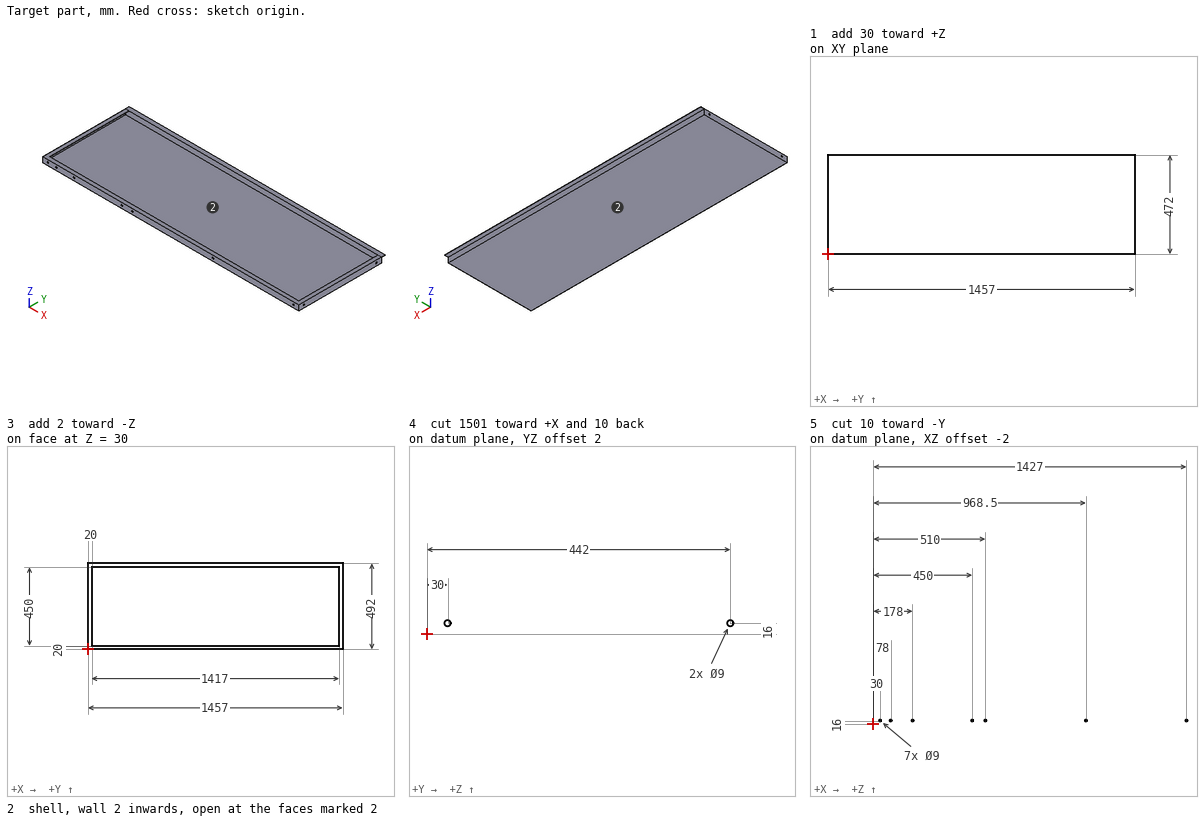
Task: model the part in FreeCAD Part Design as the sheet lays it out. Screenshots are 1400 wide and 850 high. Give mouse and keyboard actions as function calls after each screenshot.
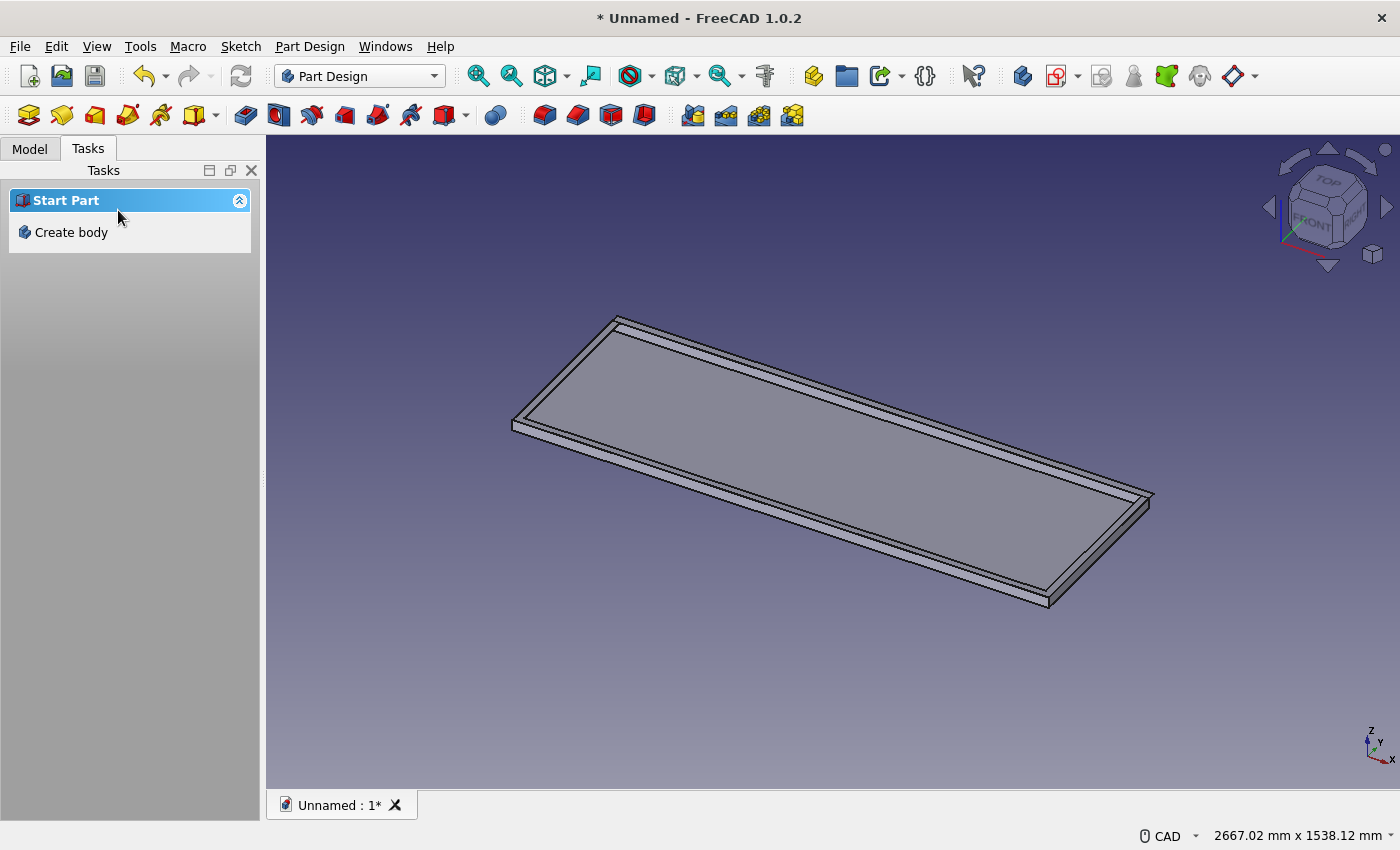
click(30, 148)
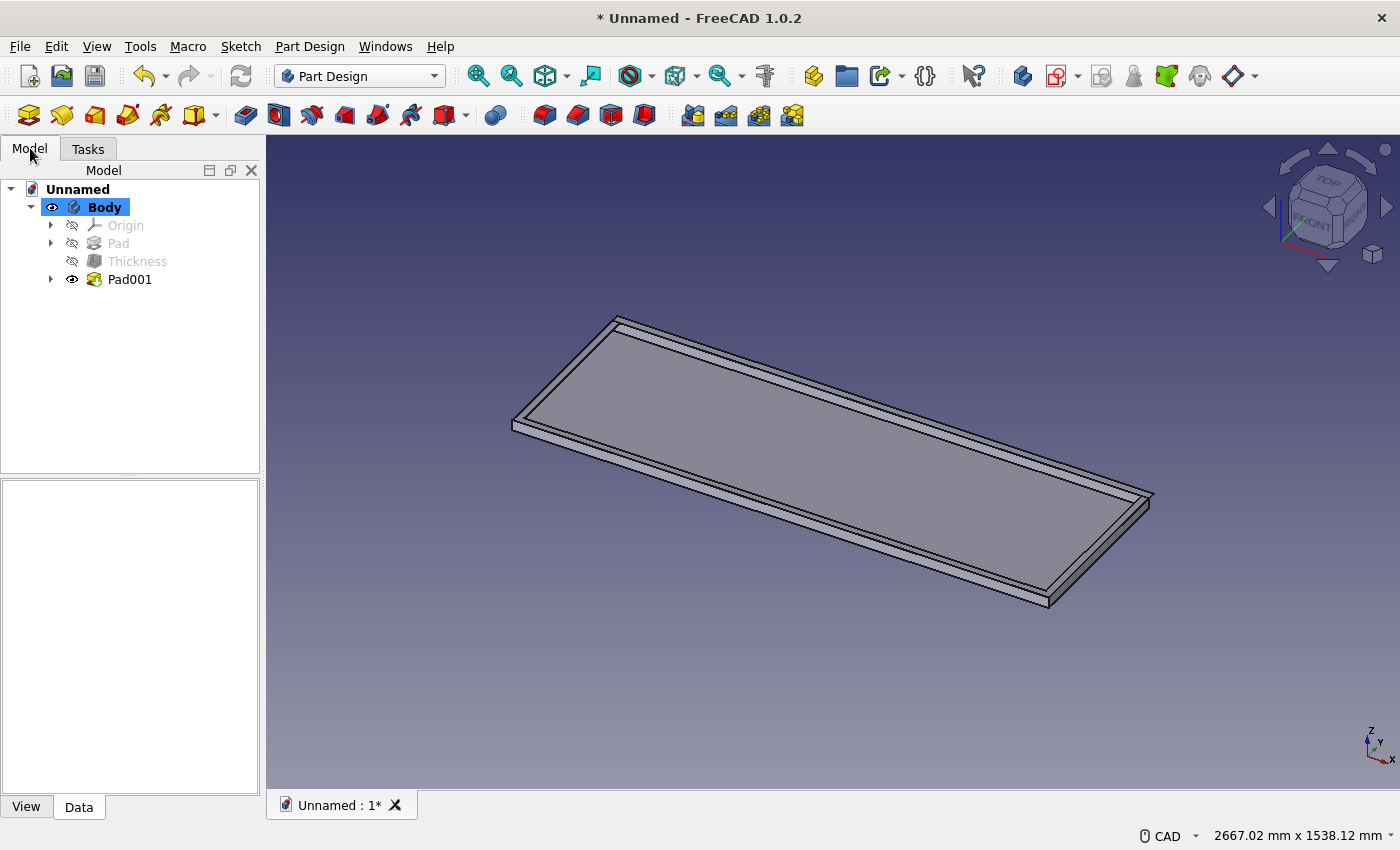
click(51, 225)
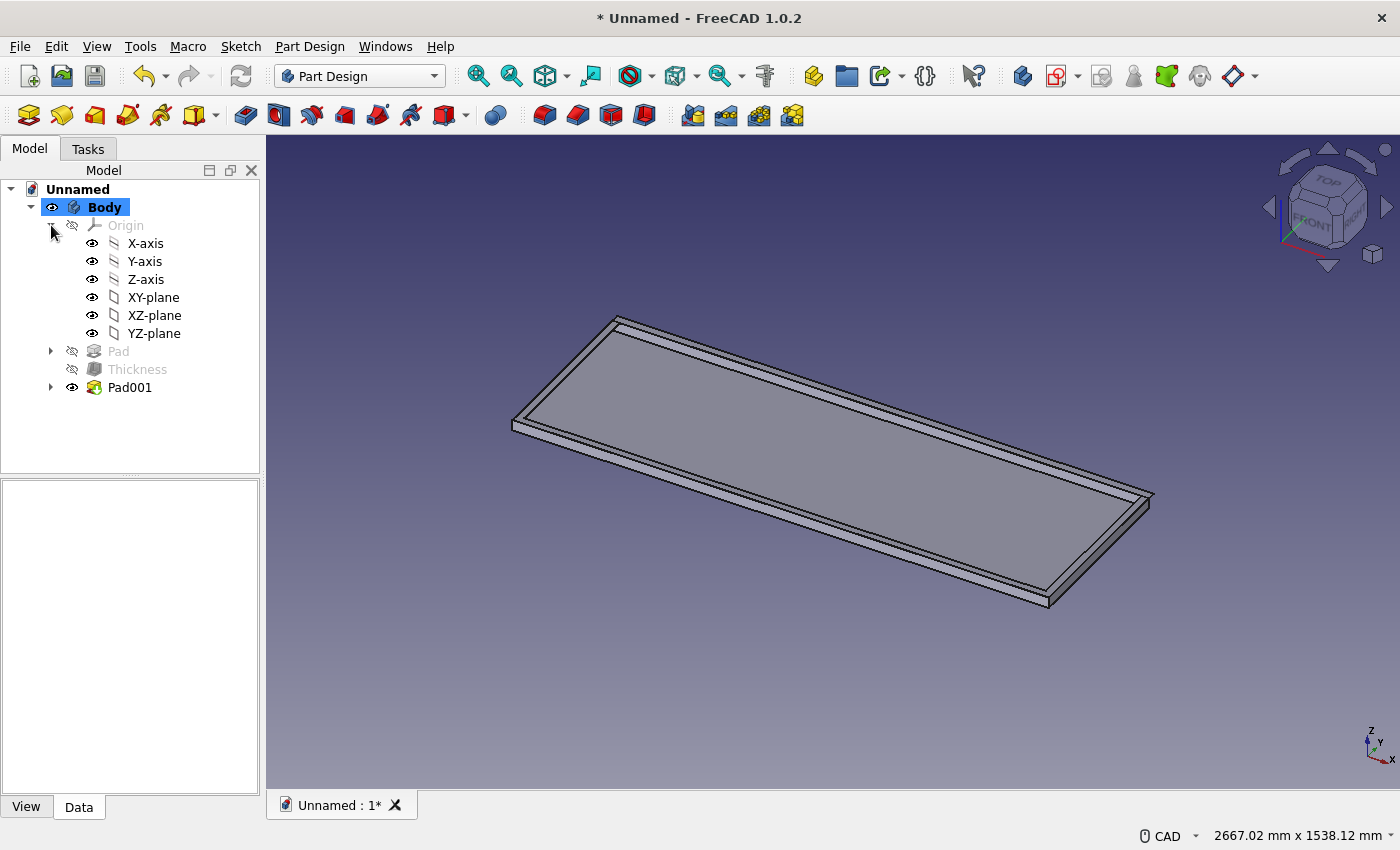
click(137, 333)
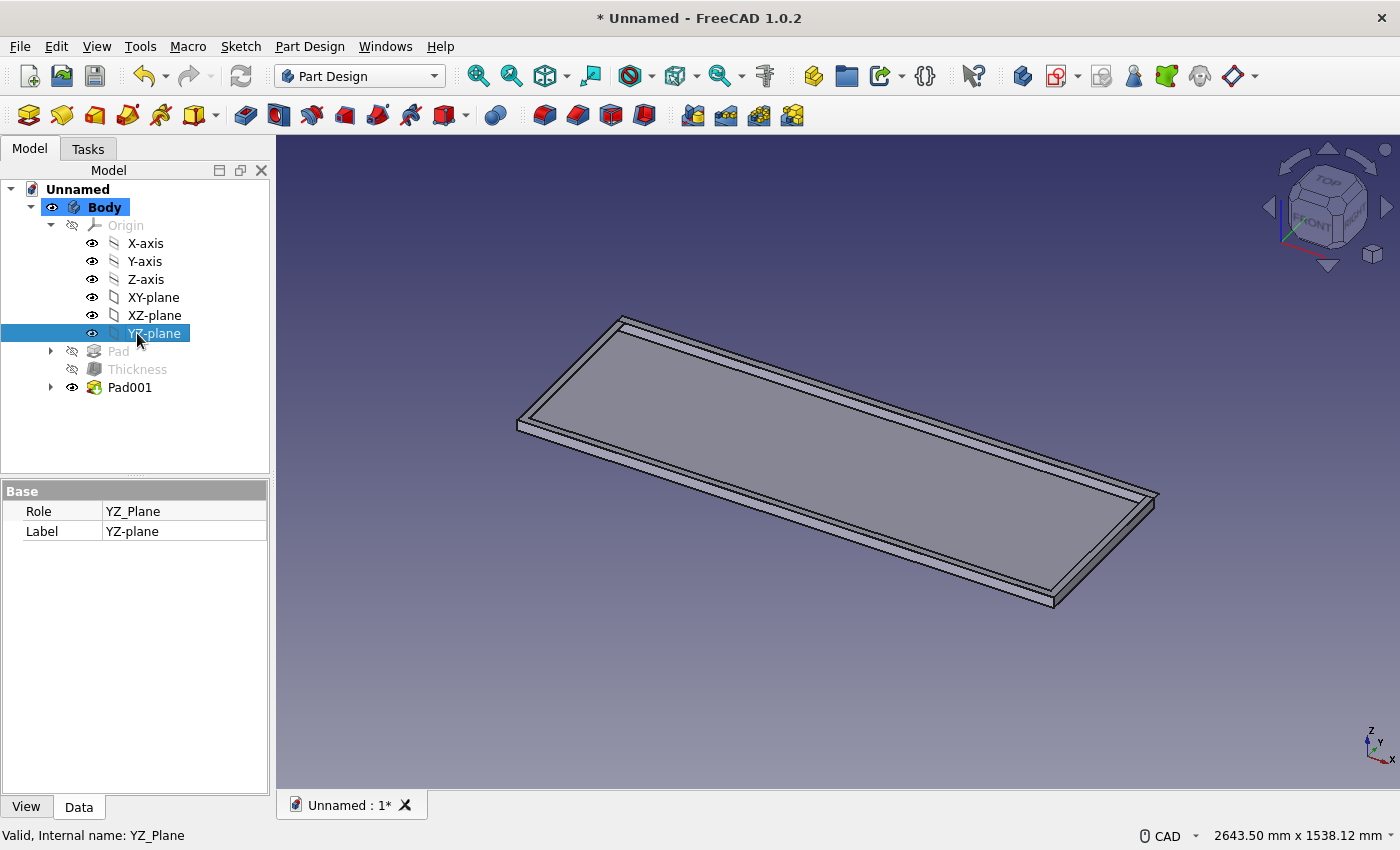
click(1232, 76)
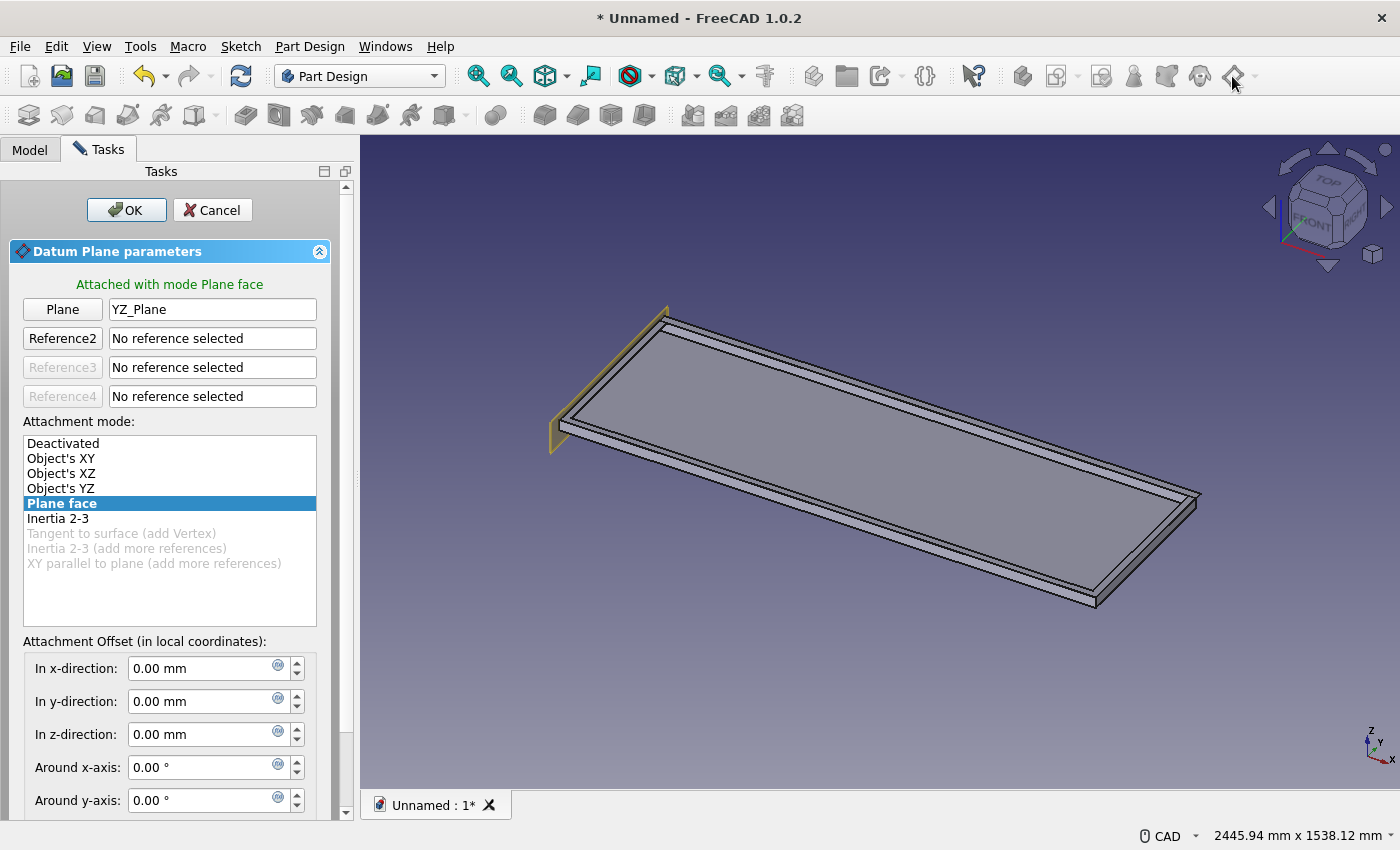
triple_click(210, 734)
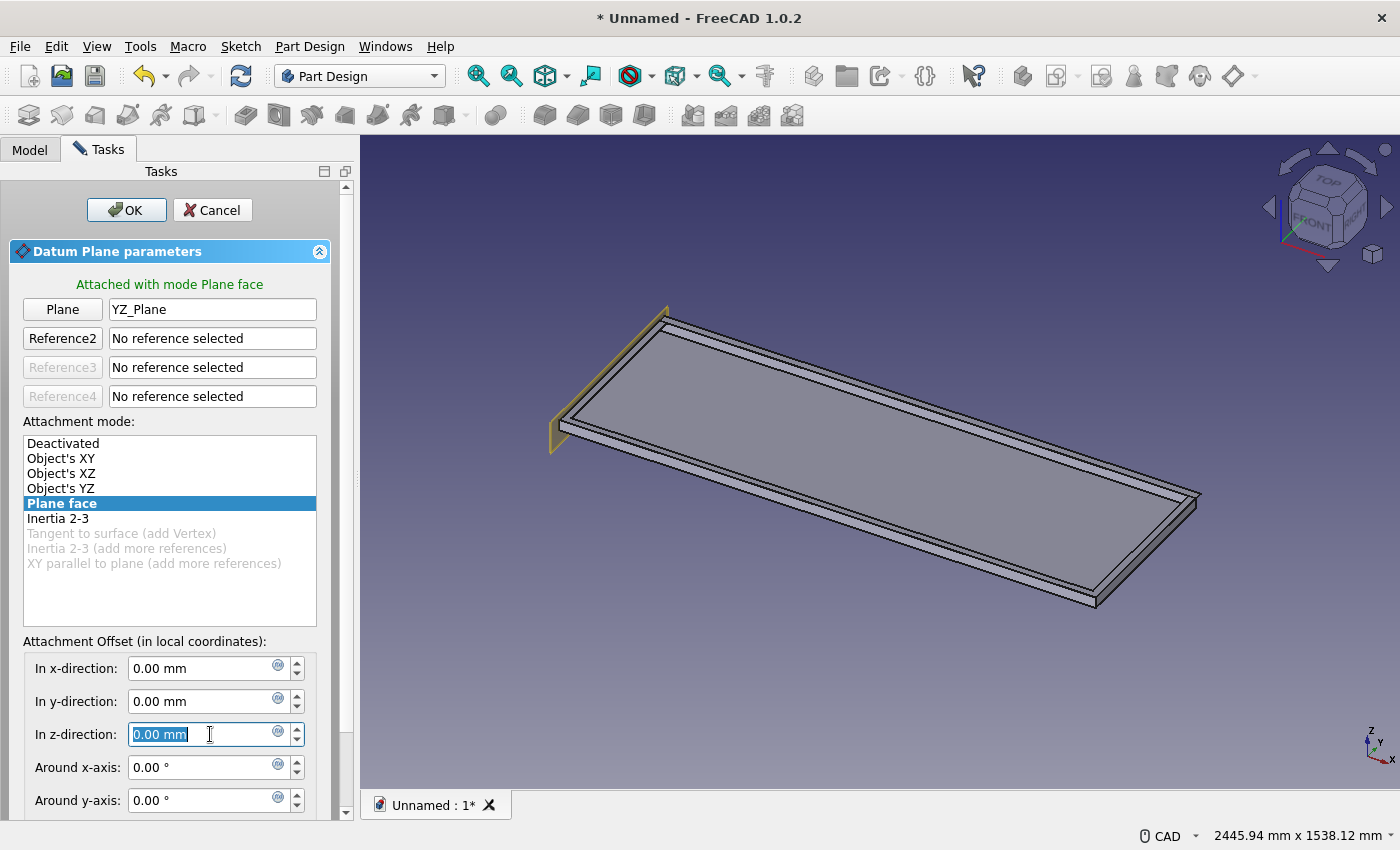
text(2)
key(Tab)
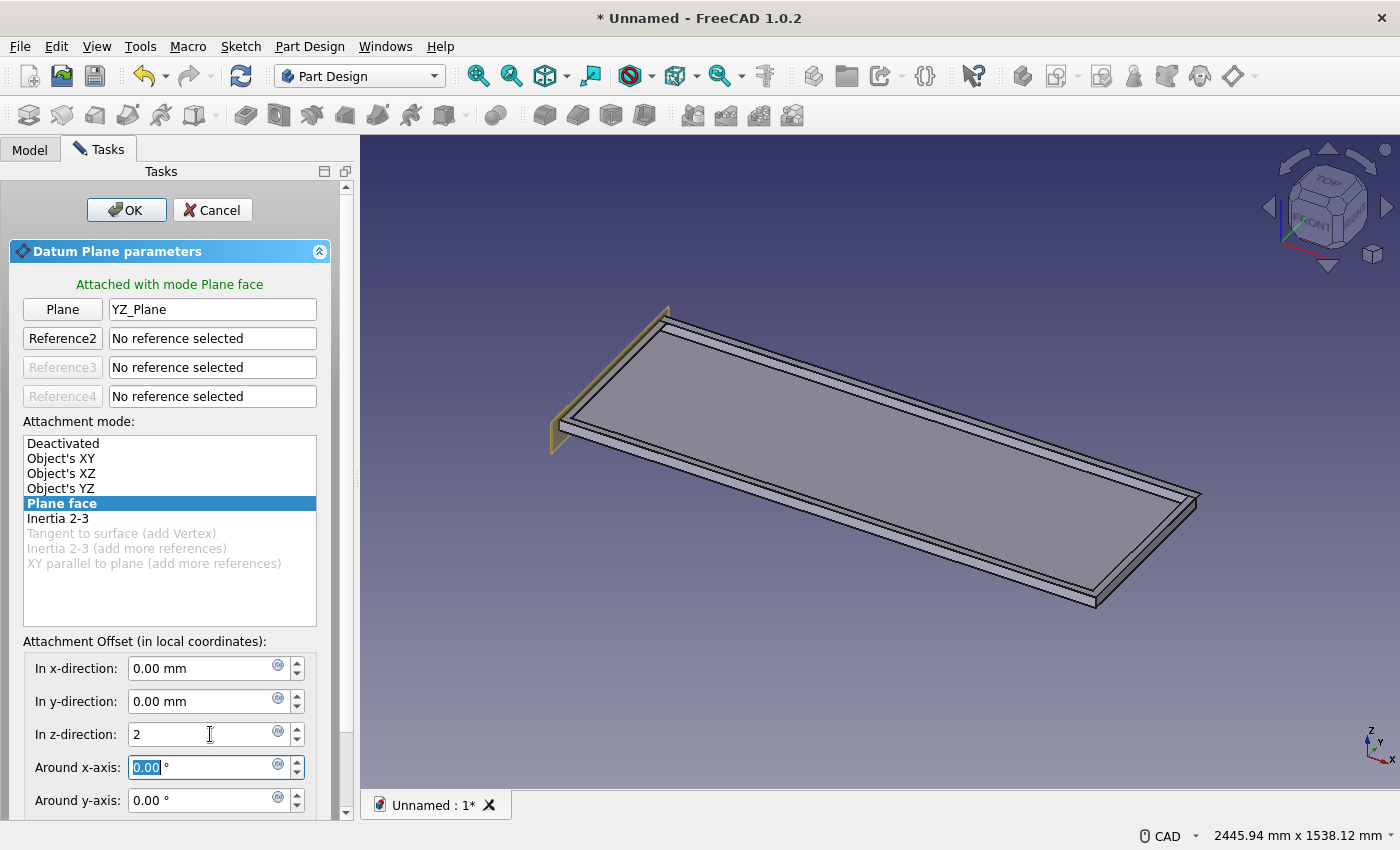
click(127, 210)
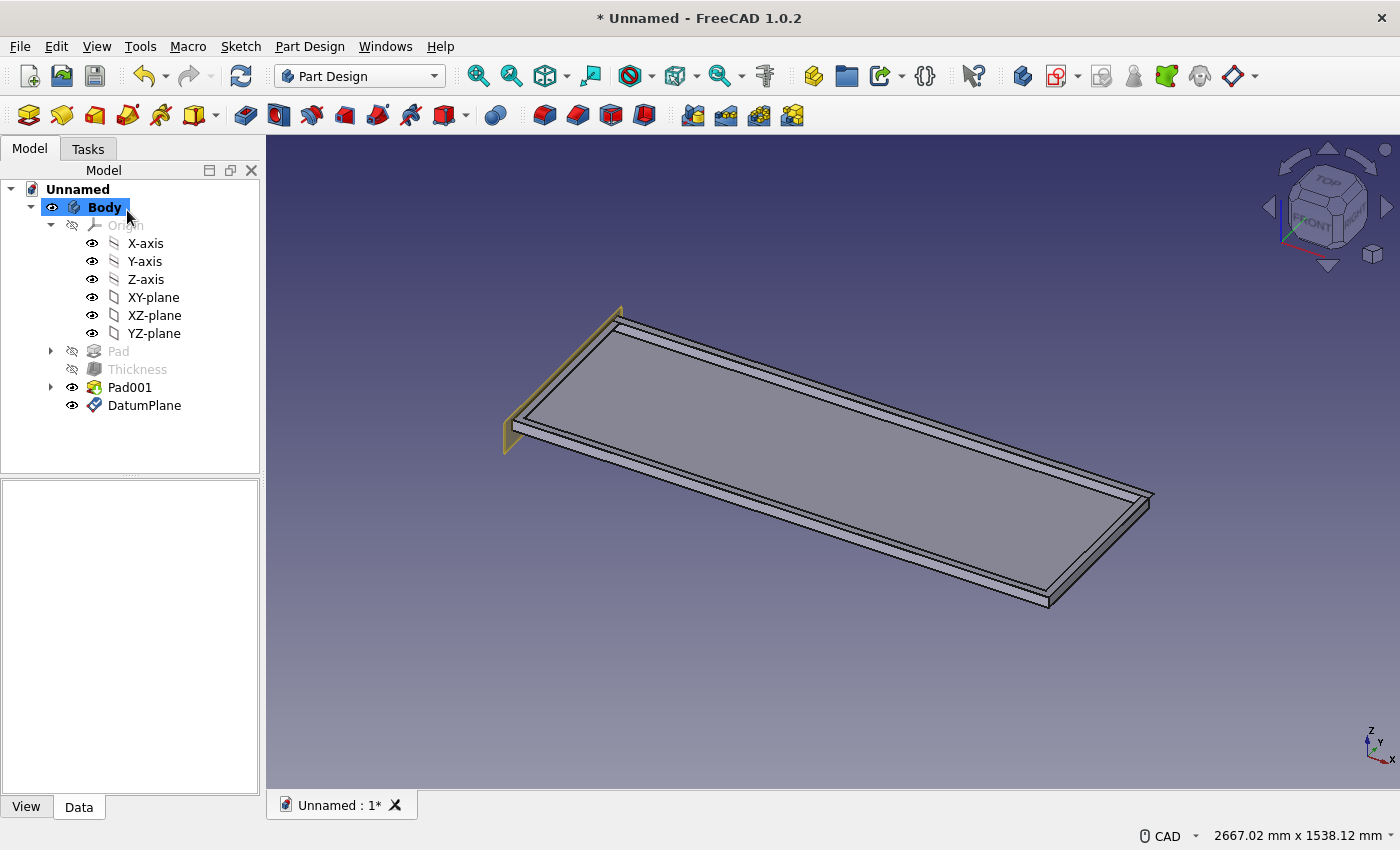
click(117, 405)